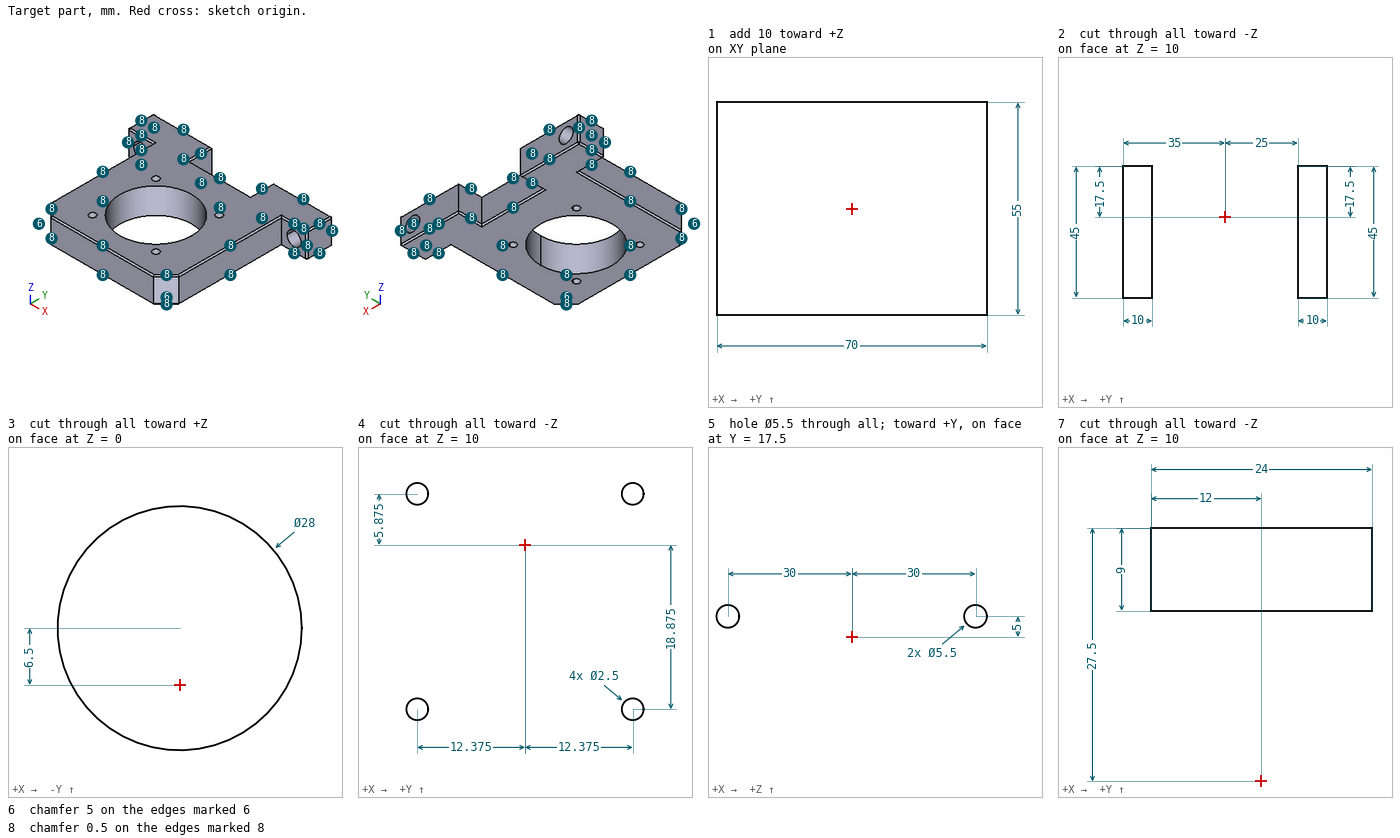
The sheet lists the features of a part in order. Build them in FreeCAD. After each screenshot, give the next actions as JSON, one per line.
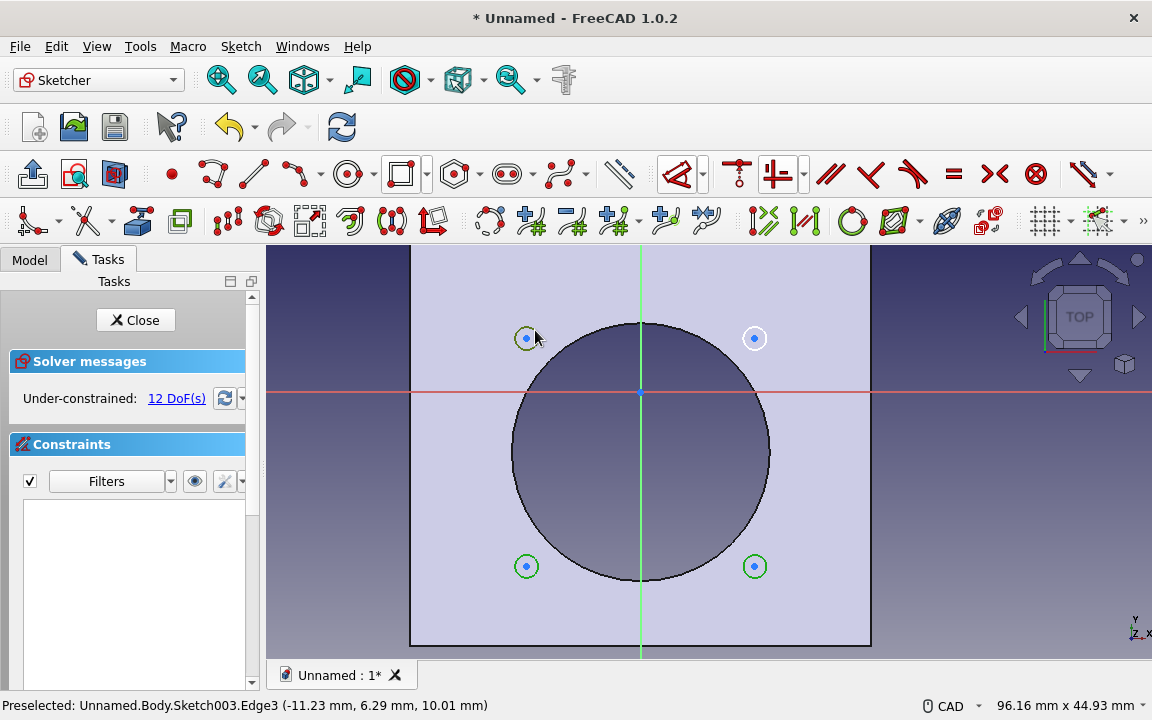
{"action": "left_click", "coordinate": [763, 330]}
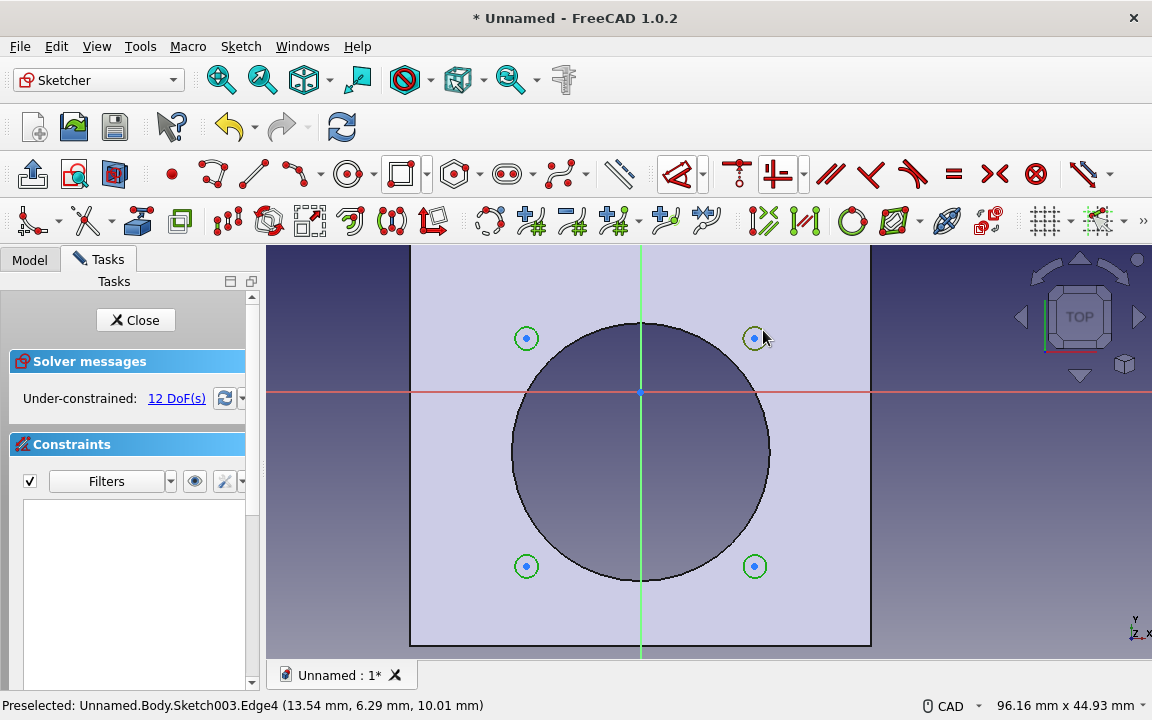
{"action": "left_click", "coordinate": [954, 174]}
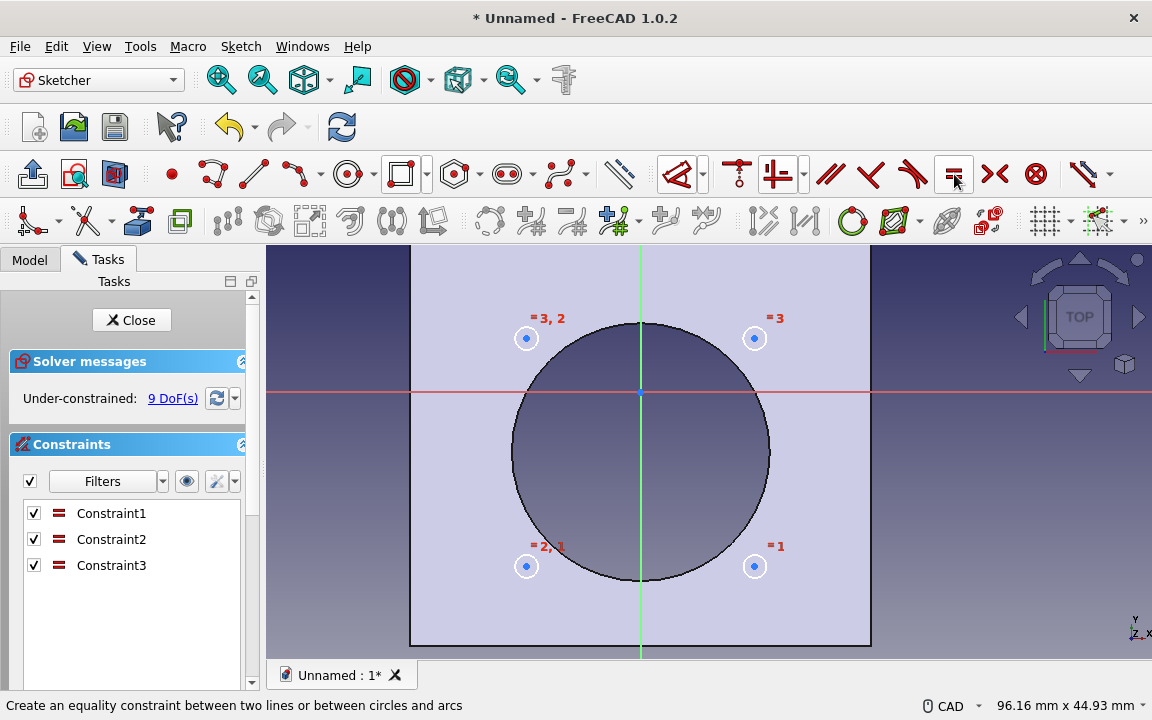
{"action": "left_click", "coordinate": [755, 567]}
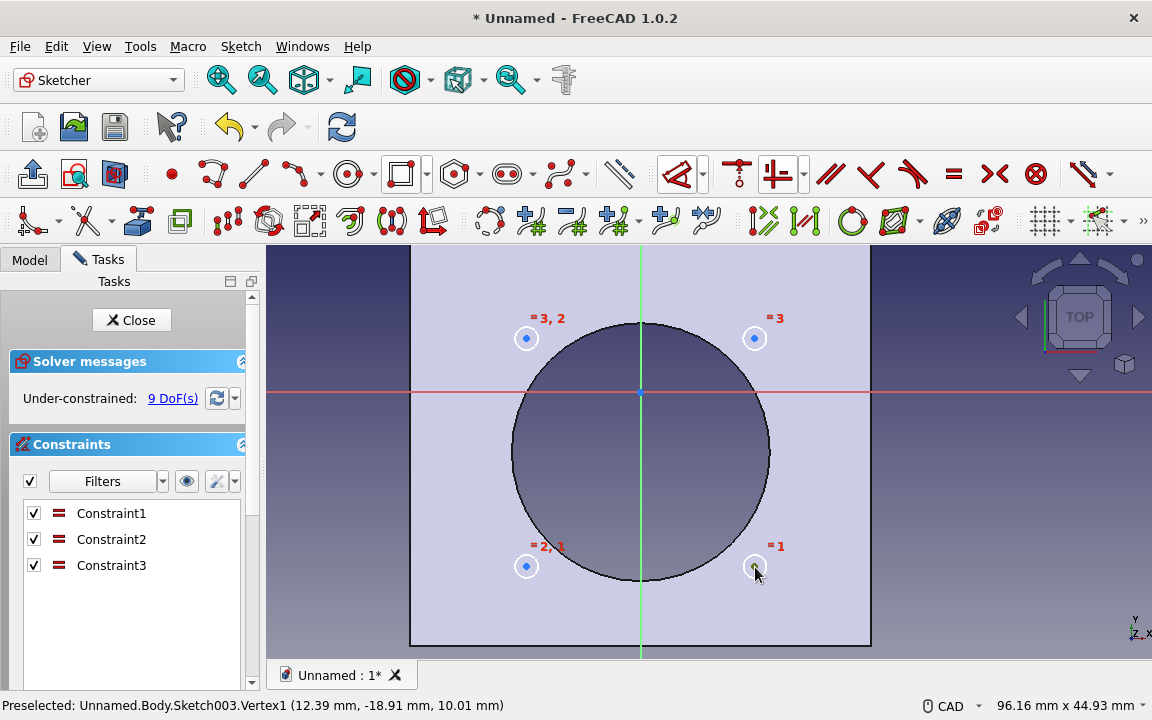
{"action": "left_click", "coordinate": [527, 566]}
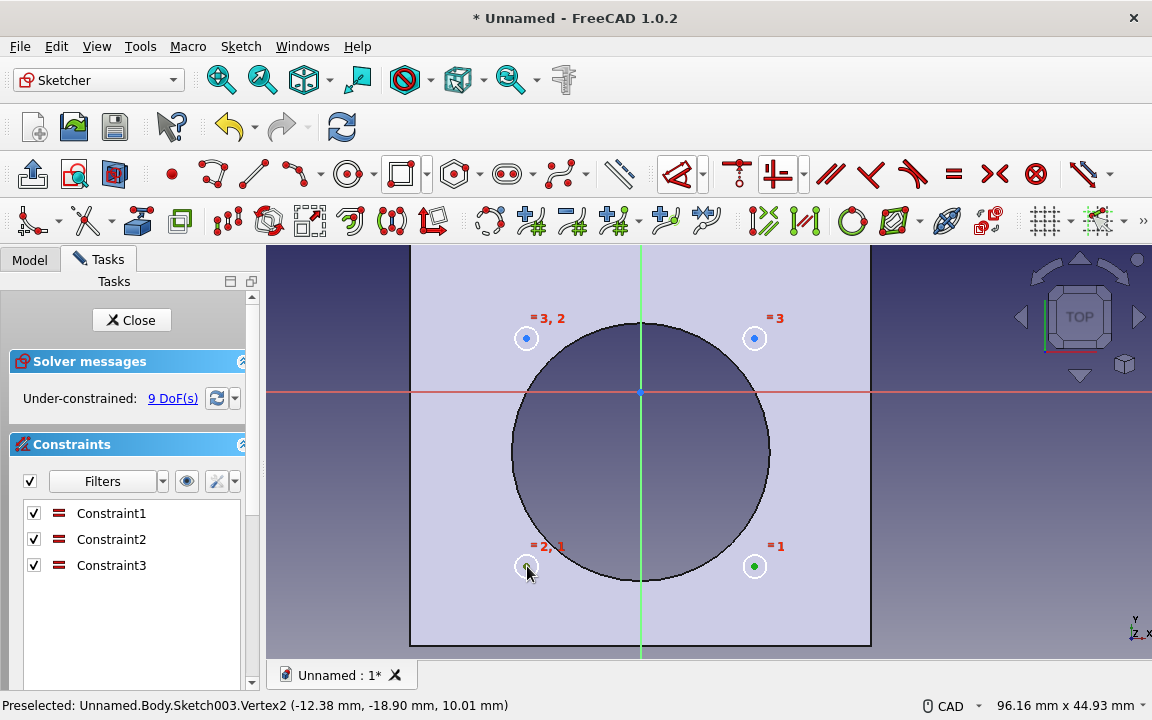
{"action": "left_click", "coordinate": [804, 174]}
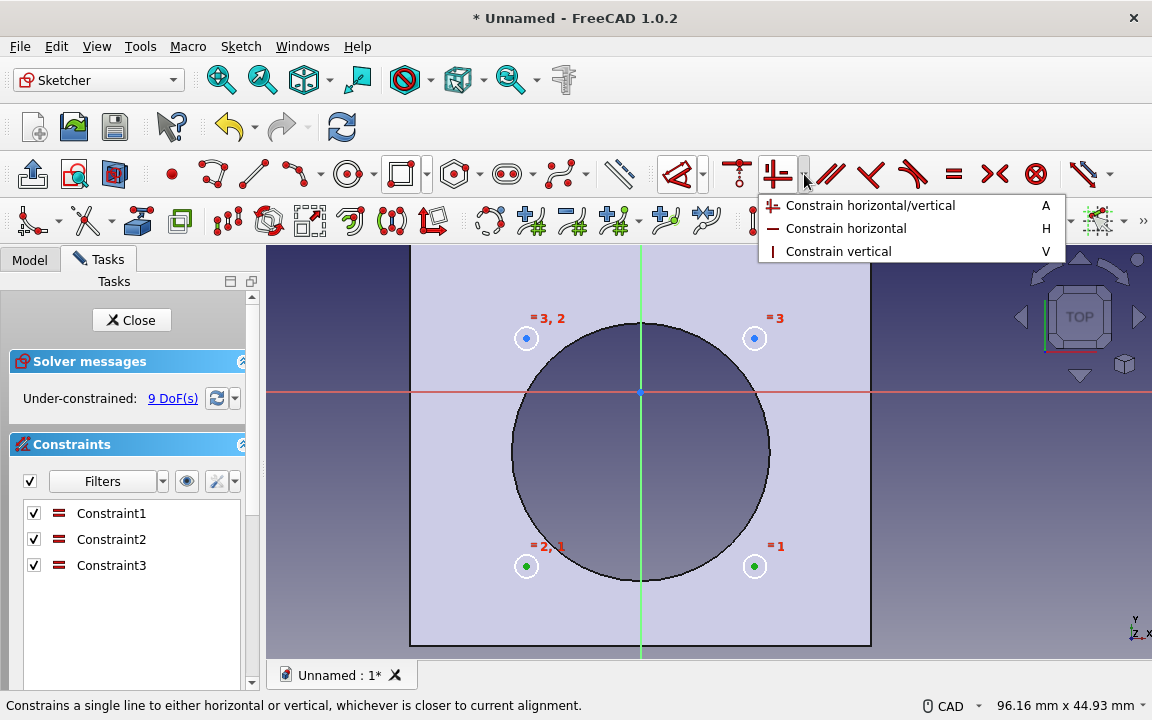
{"action": "left_click", "coordinate": [912, 228]}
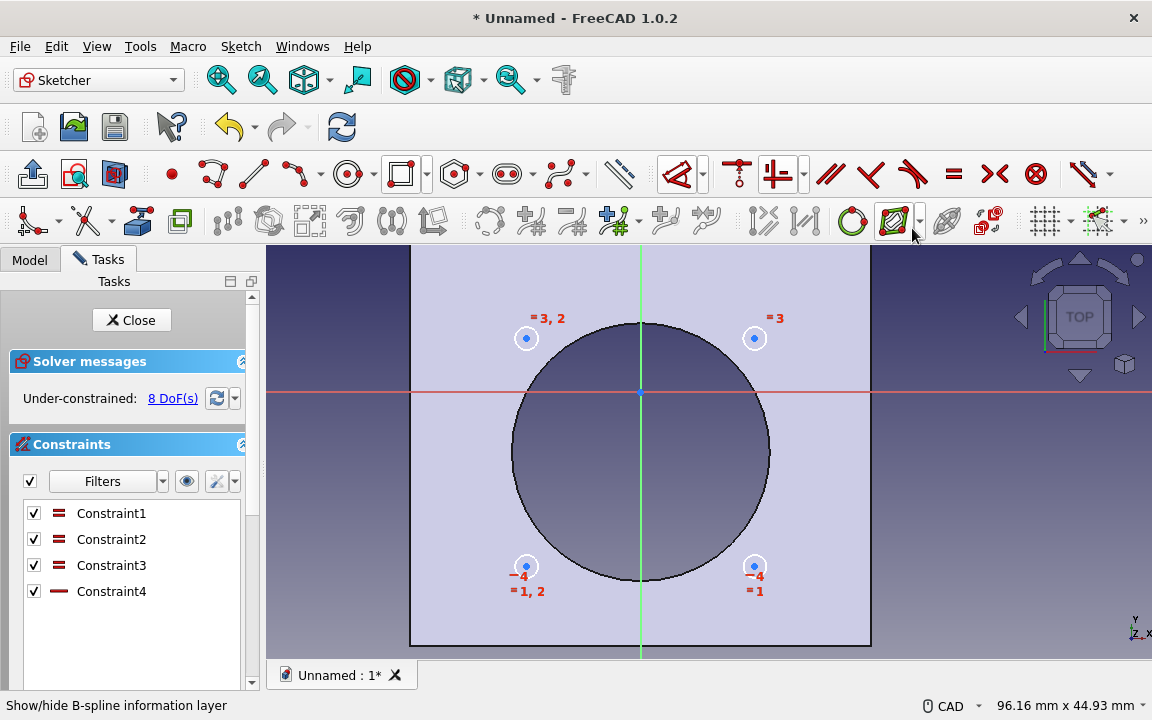
{"action": "left_click", "coordinate": [527, 567]}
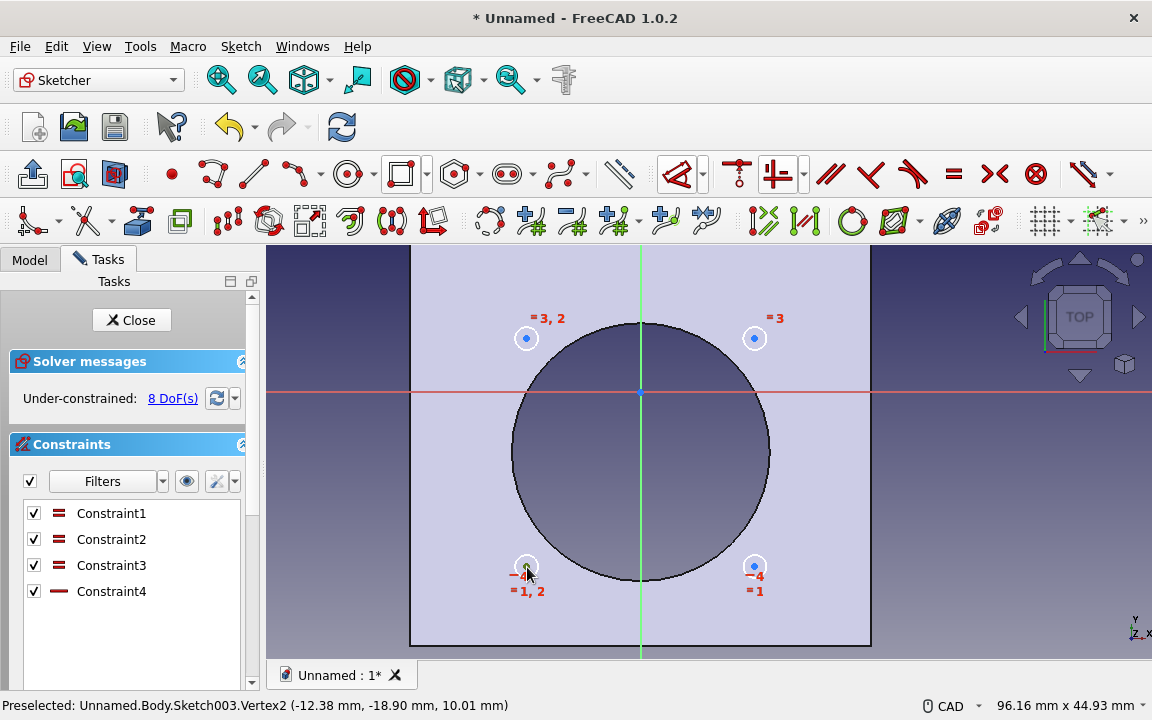
{"action": "left_click", "coordinate": [527, 339]}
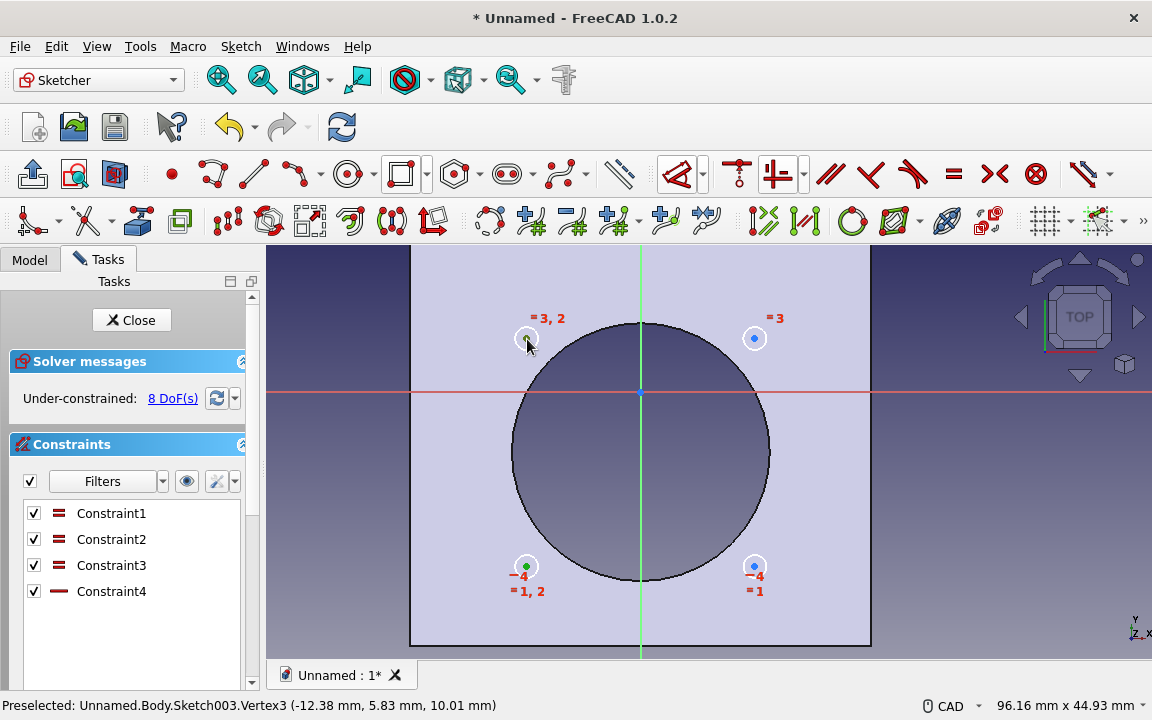
{"action": "left_click", "coordinate": [804, 174]}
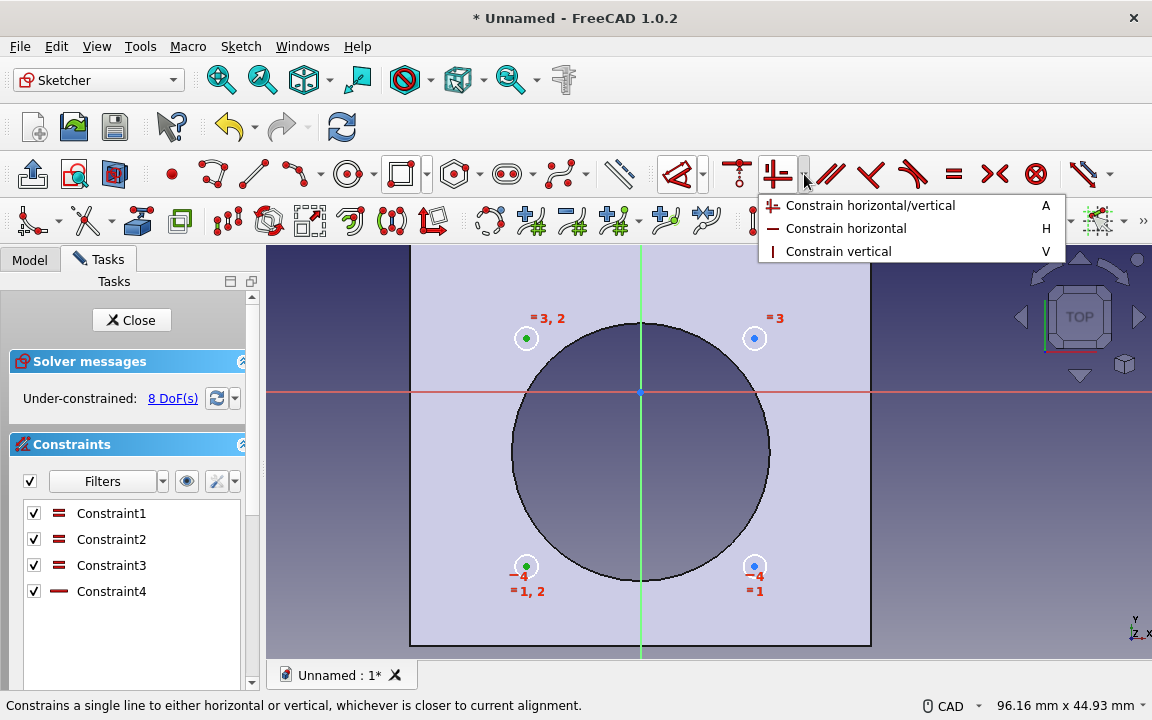
{"action": "left_click", "coordinate": [912, 252]}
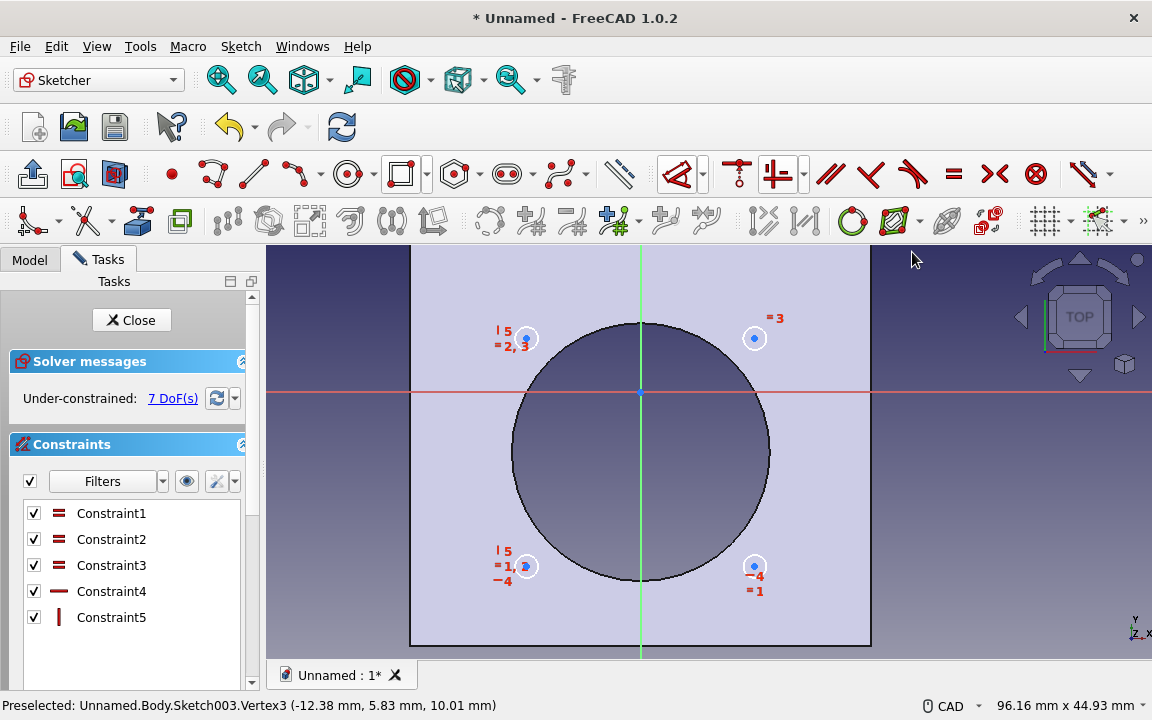
{"action": "left_click", "coordinate": [755, 567]}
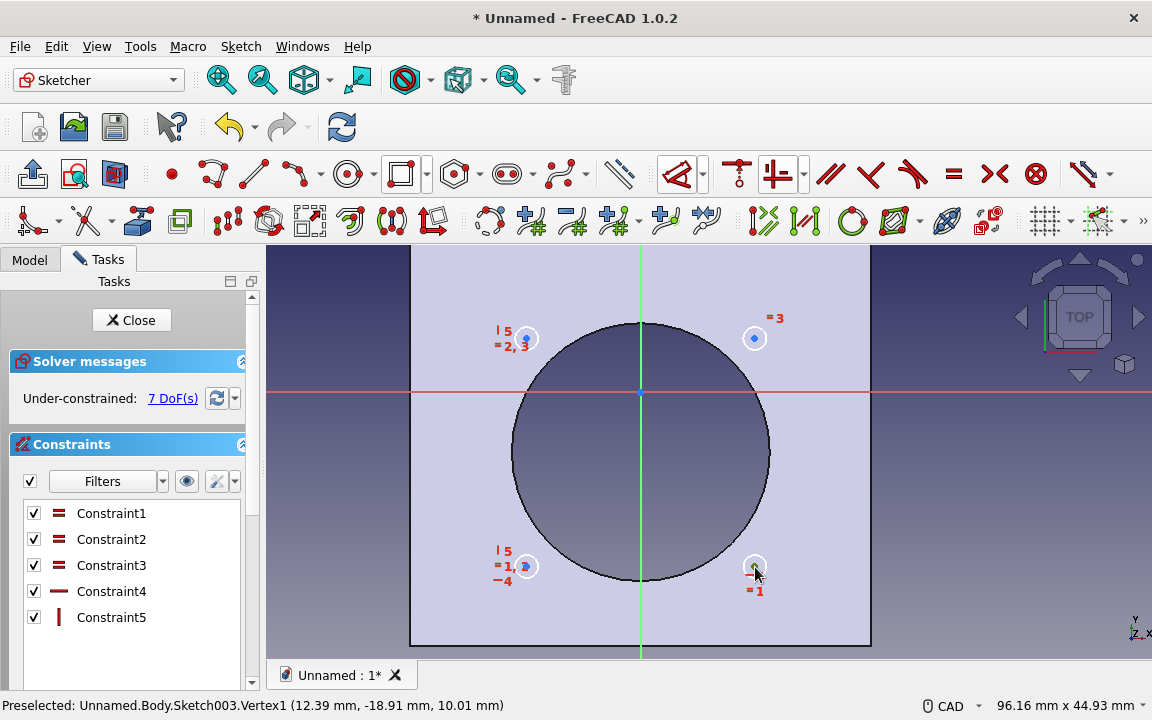
{"action": "left_click", "coordinate": [755, 339]}